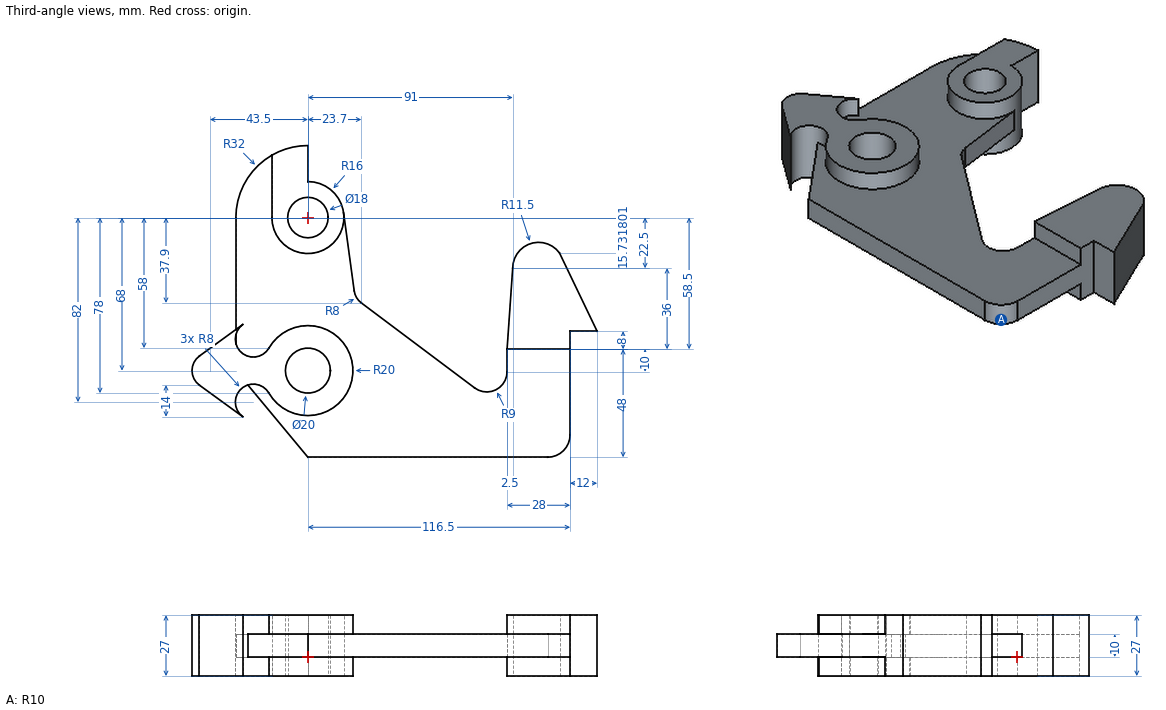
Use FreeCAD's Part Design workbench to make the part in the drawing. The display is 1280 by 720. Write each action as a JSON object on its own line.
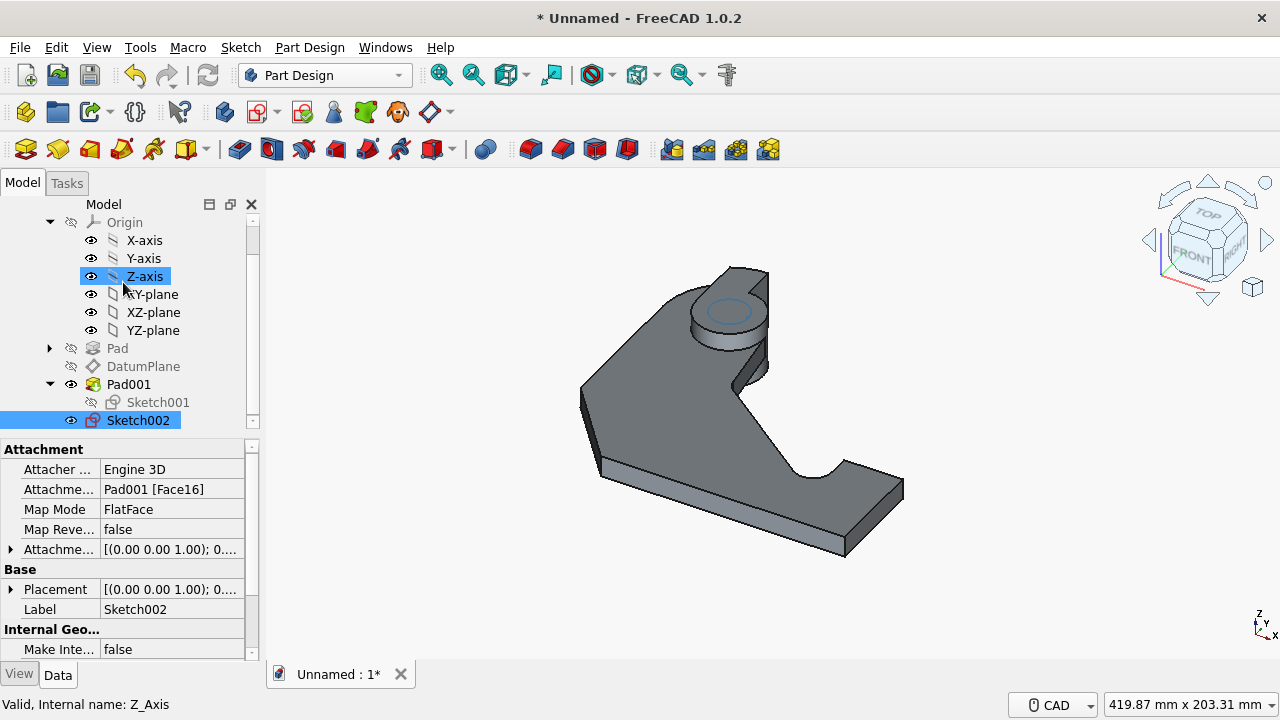
{"action": "left_click", "coordinate": [240, 150]}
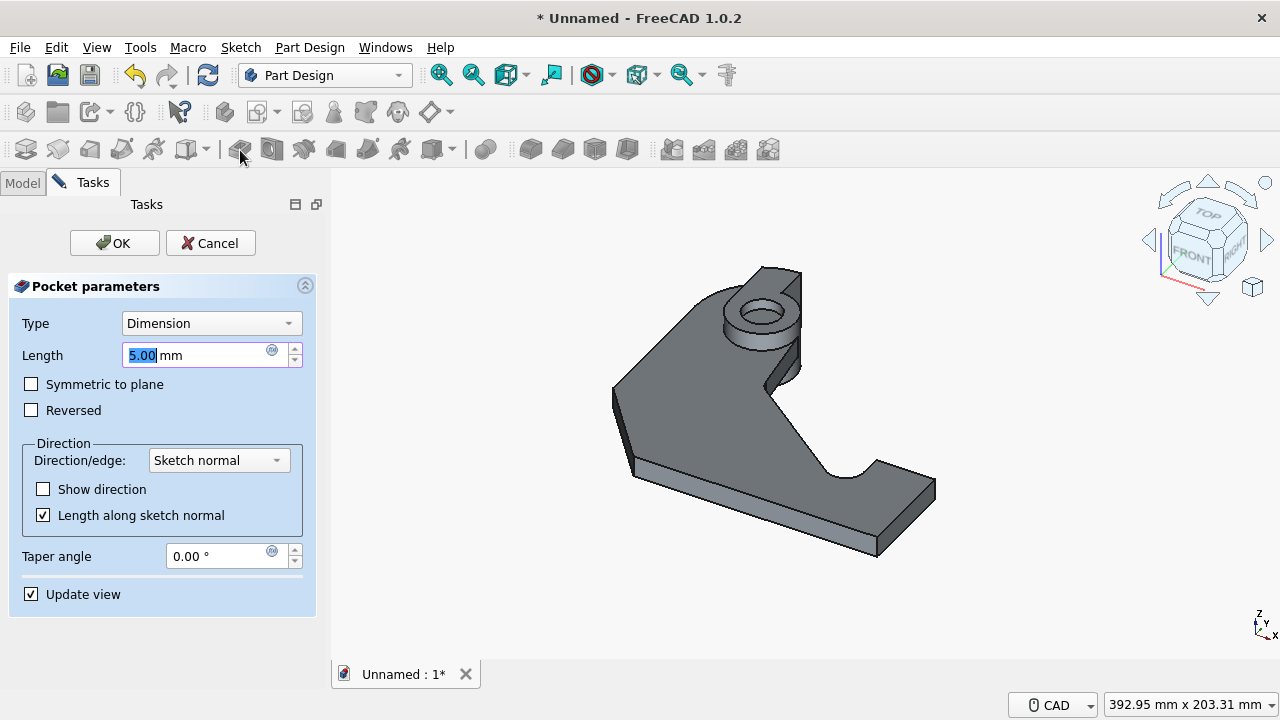
{"action": "type", "text": "27"}
{"action": "key", "text": "Tab"}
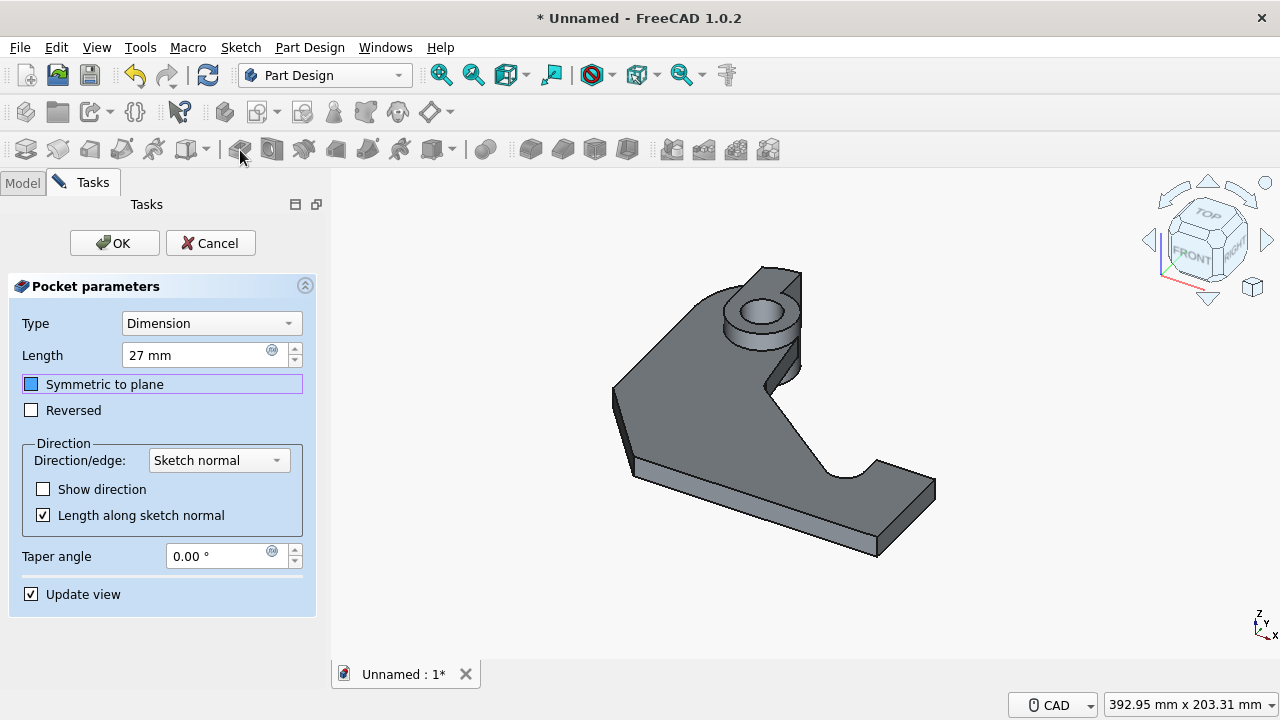
{"action": "left_click", "coordinate": [115, 243]}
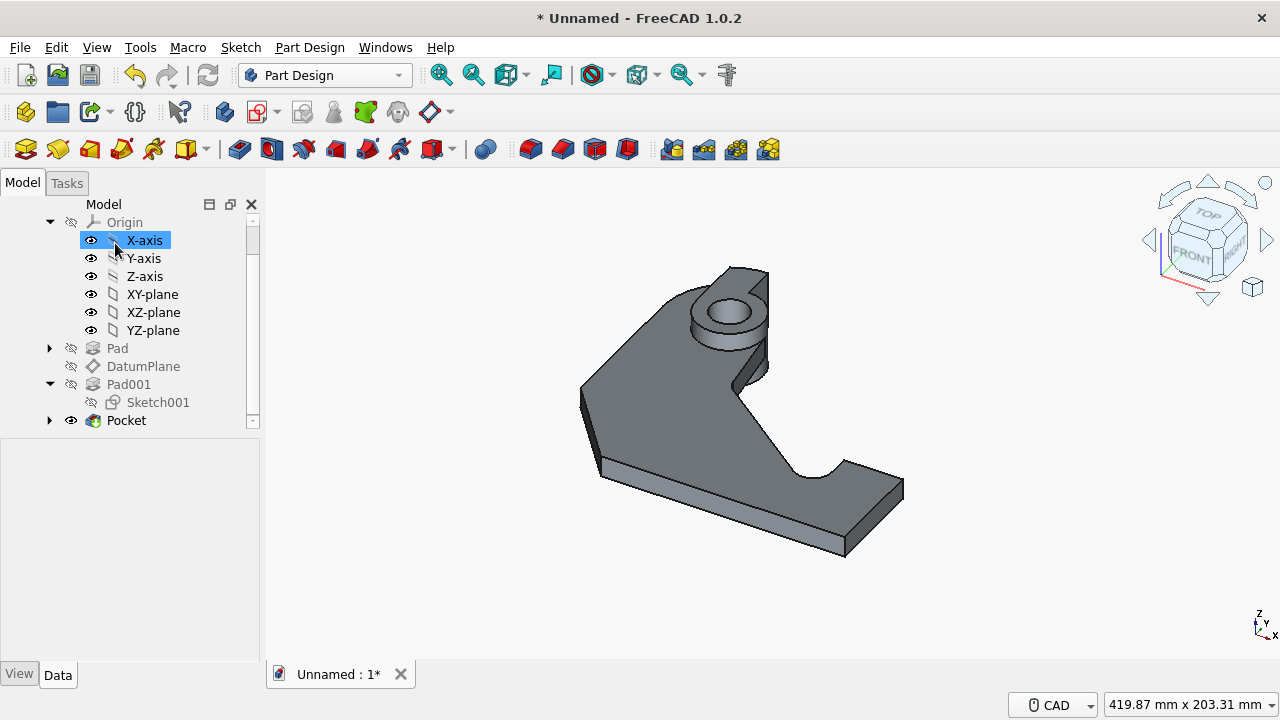
{"action": "left_click", "coordinate": [136, 294]}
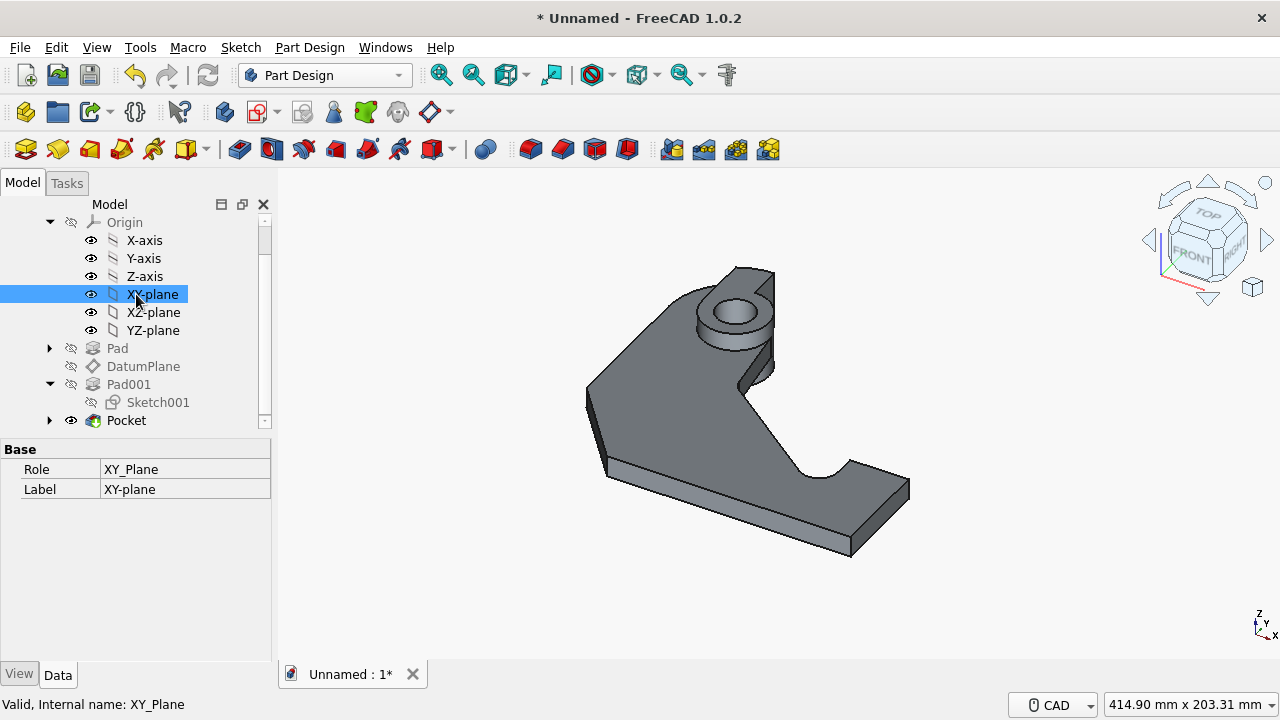
{"action": "left_click", "coordinate": [430, 112]}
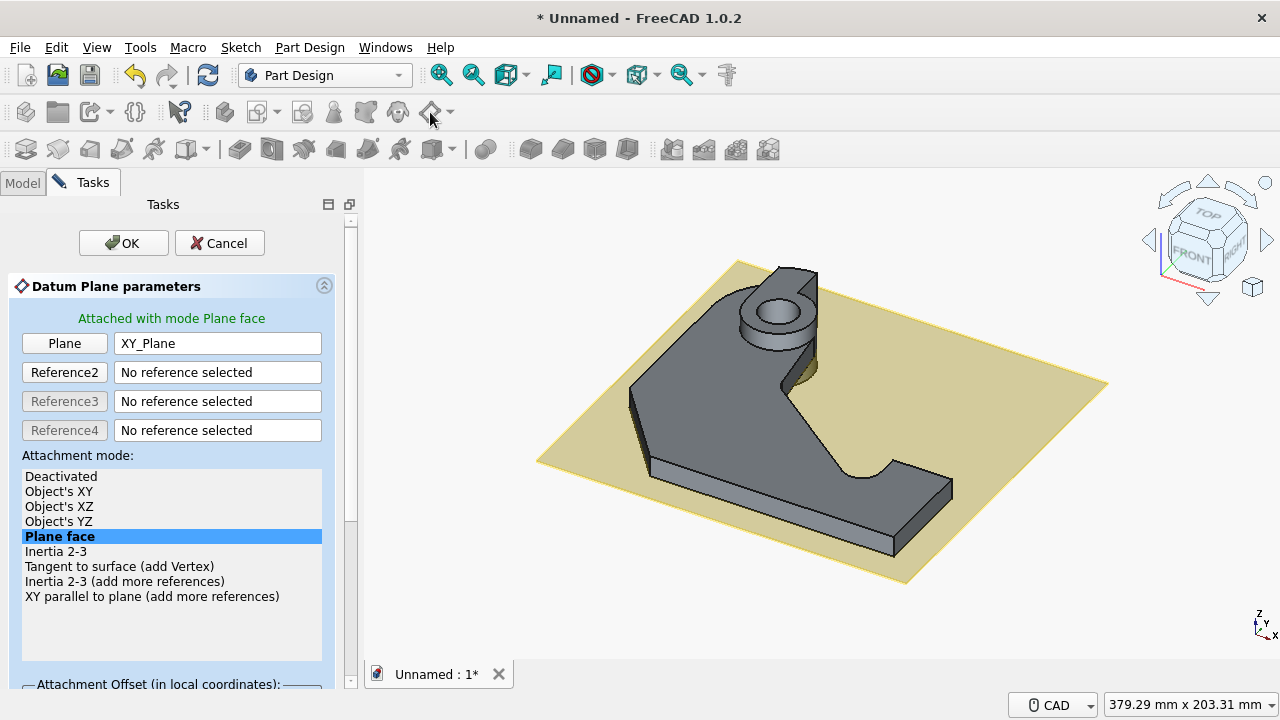
{"action": "scroll", "coordinate": [351, 451], "scroll_direction": "down", "scroll_amount": 3}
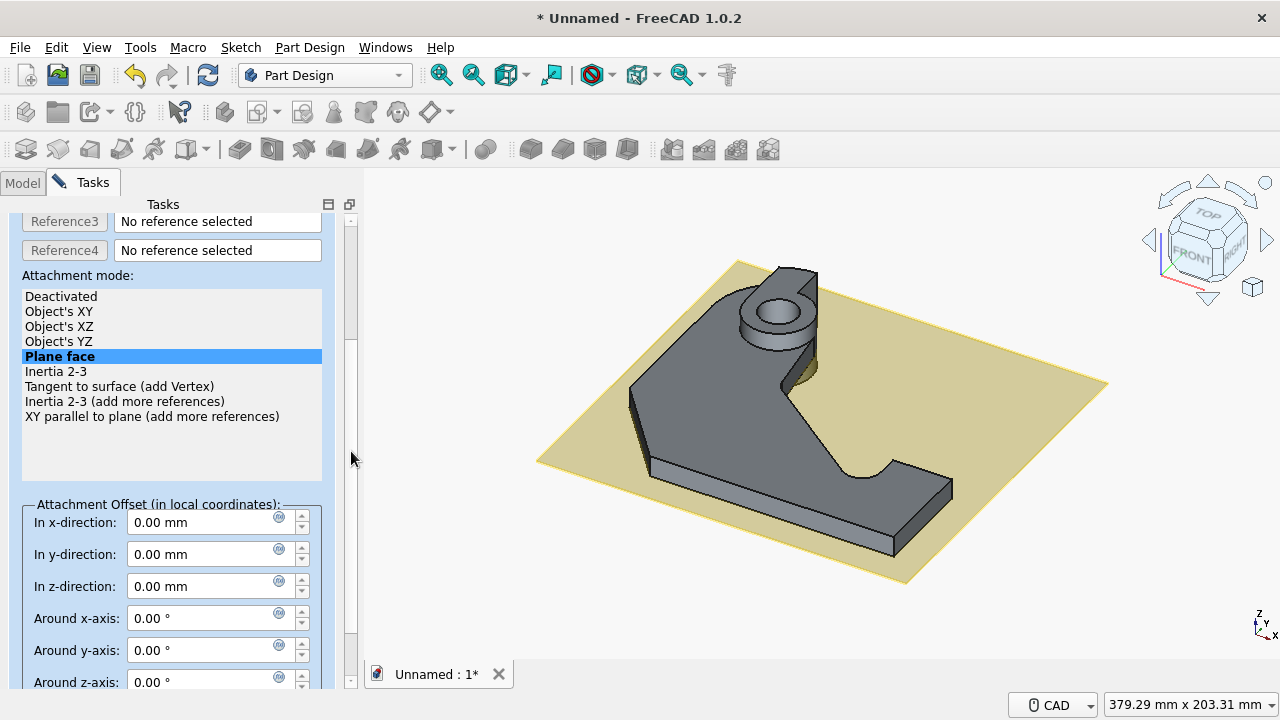
{"action": "triple_click", "coordinate": [210, 586]}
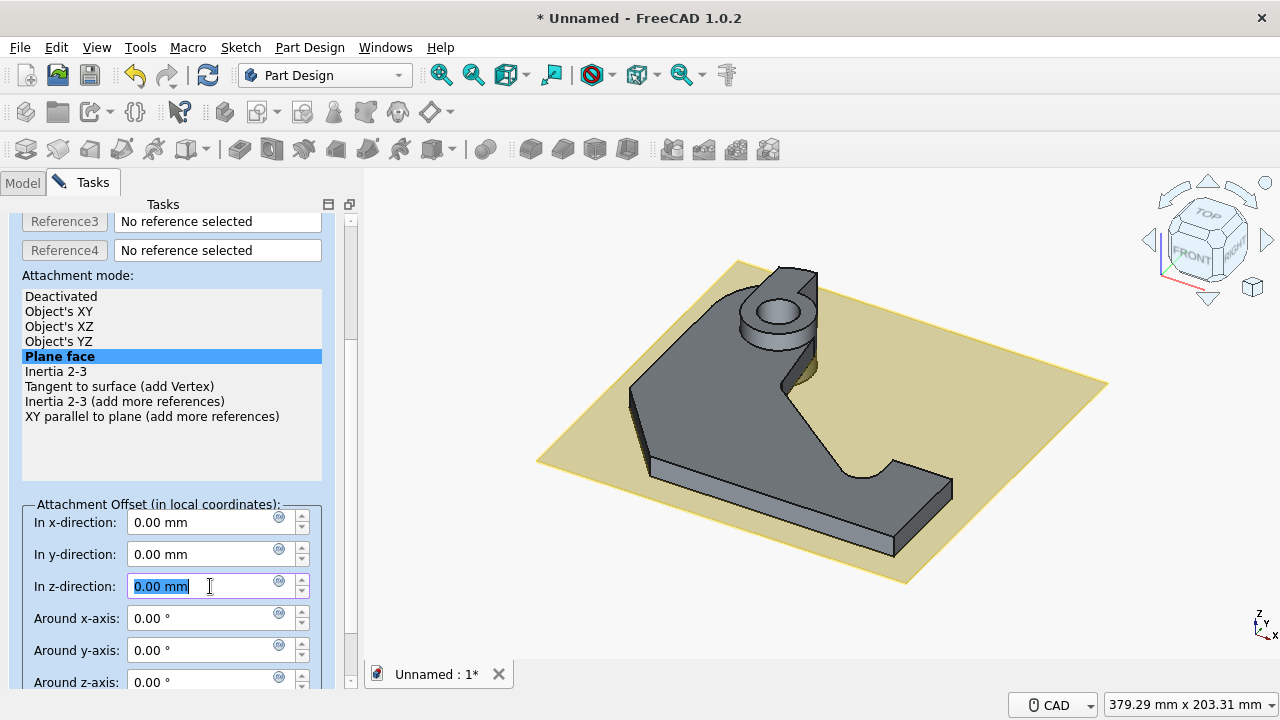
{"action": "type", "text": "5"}
{"action": "key", "text": "Tab"}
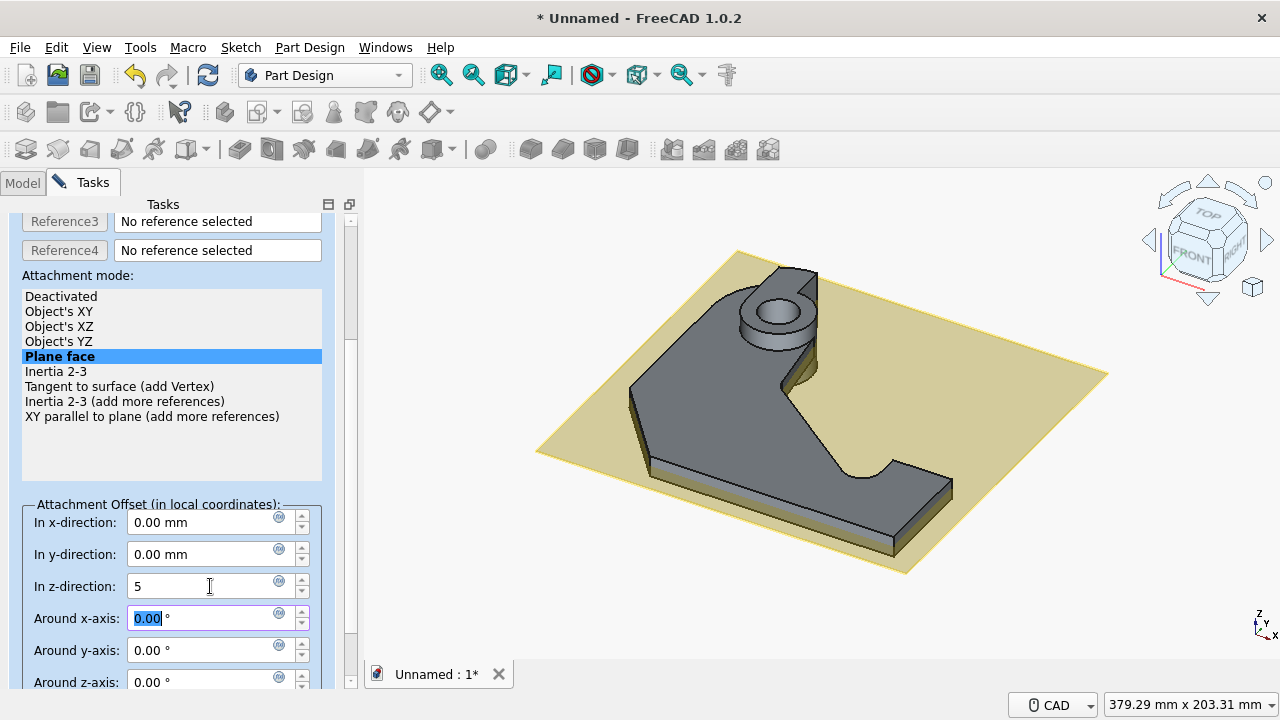
{"action": "scroll", "coordinate": [351, 451], "scroll_direction": "up", "scroll_amount": 4}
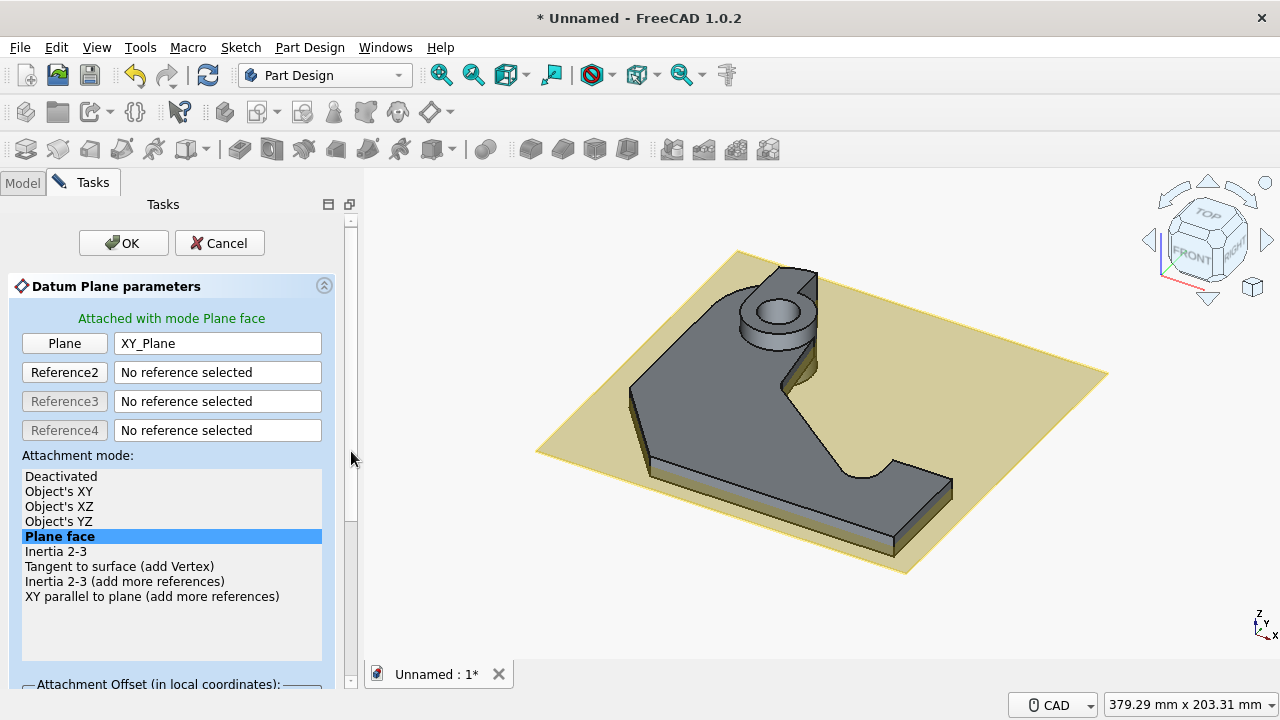
{"action": "left_click", "coordinate": [124, 243]}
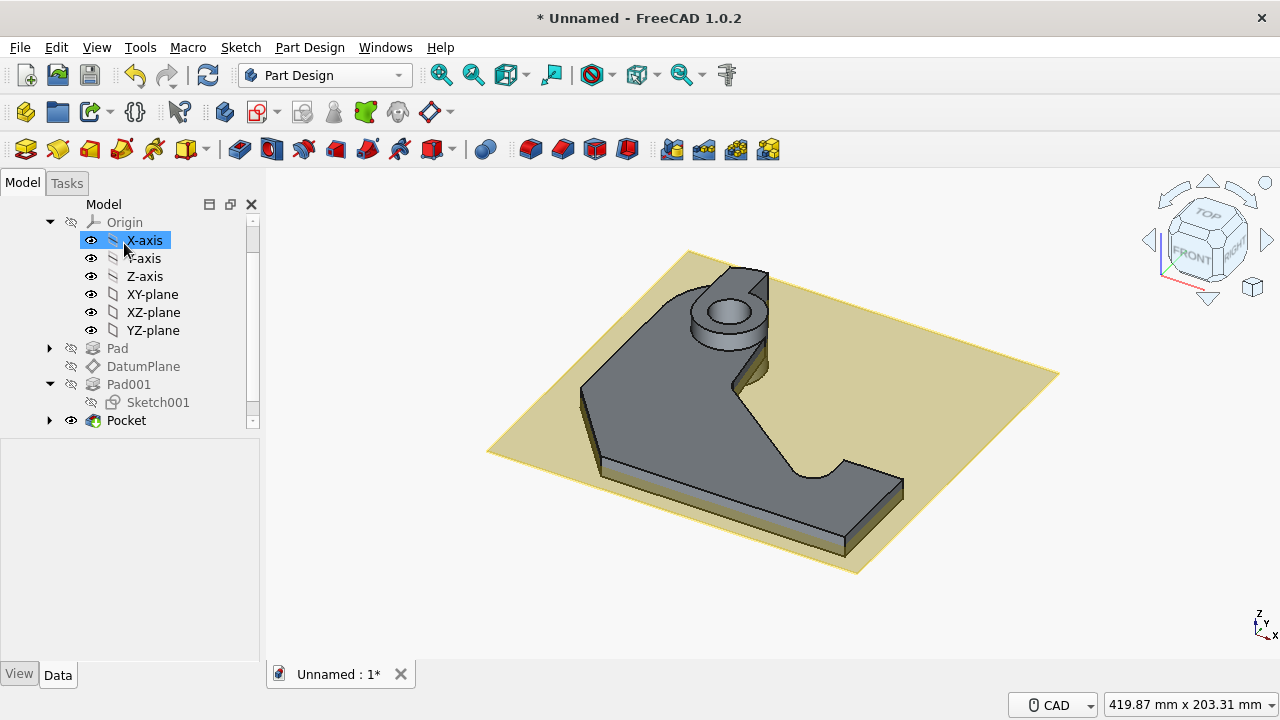
{"action": "scroll", "coordinate": [140, 326], "scroll_direction": "down", "scroll_amount": 3}